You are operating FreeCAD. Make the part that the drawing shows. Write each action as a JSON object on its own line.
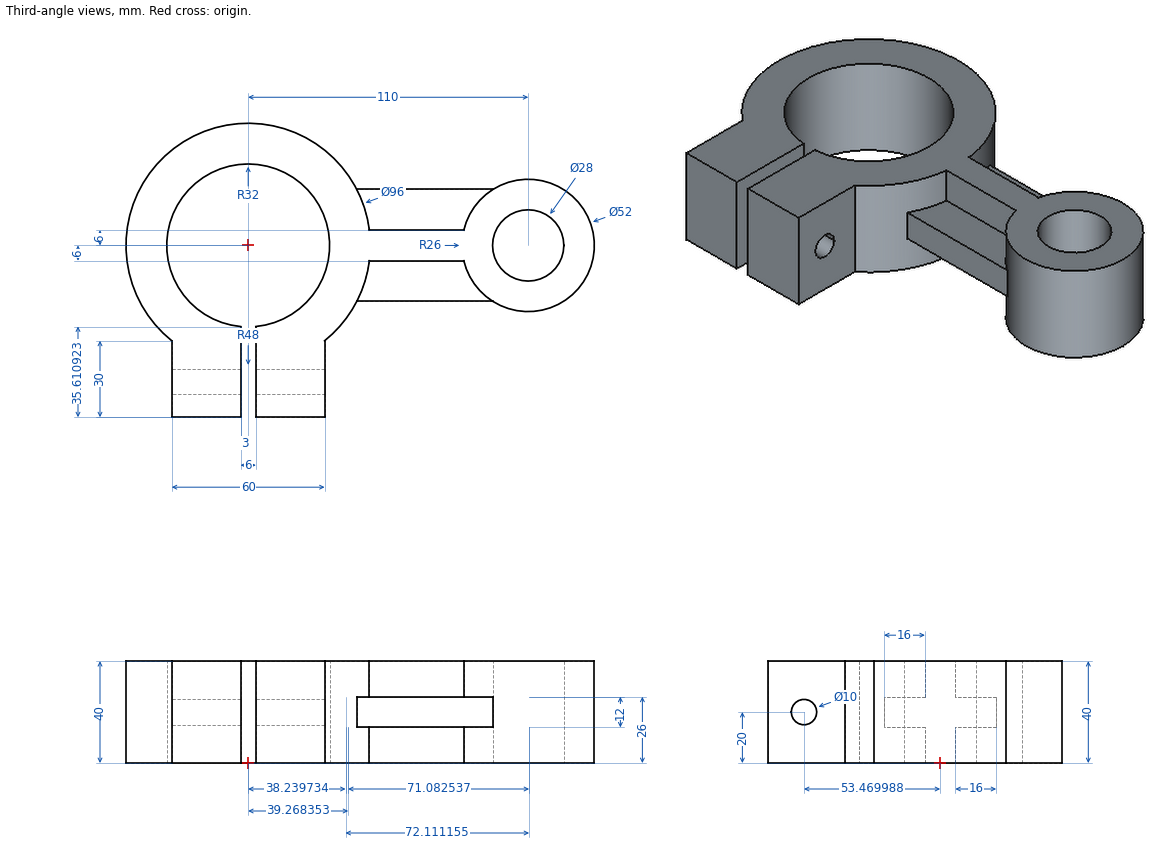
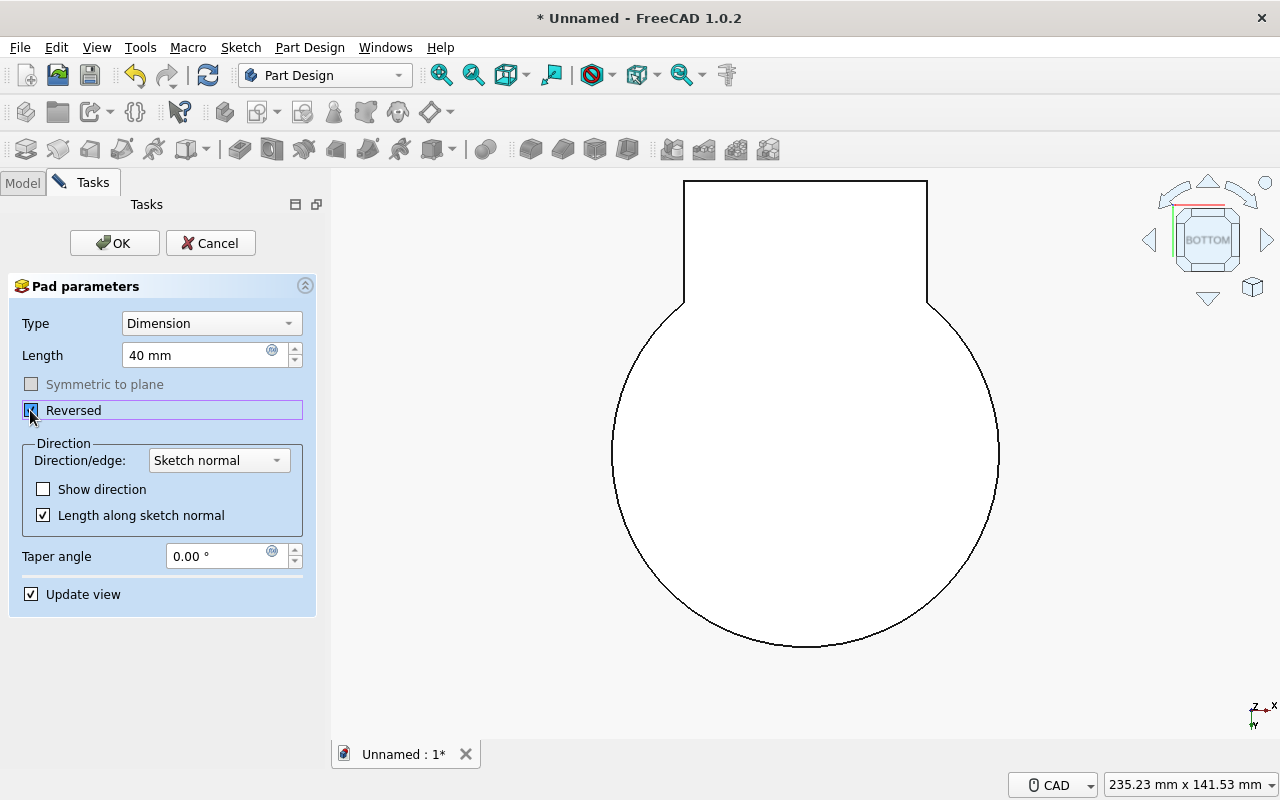
{"action": "left_click", "coordinate": [115, 243]}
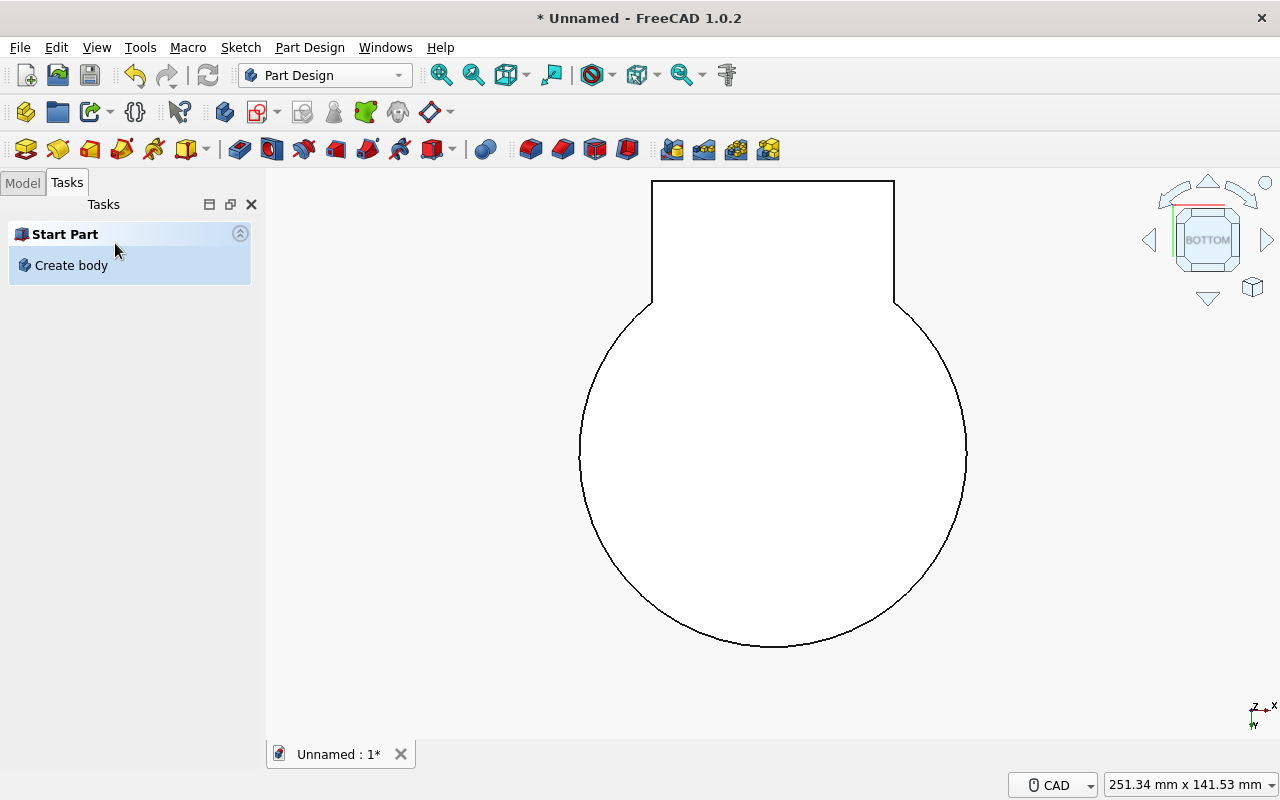
{"action": "key", "text": "0"}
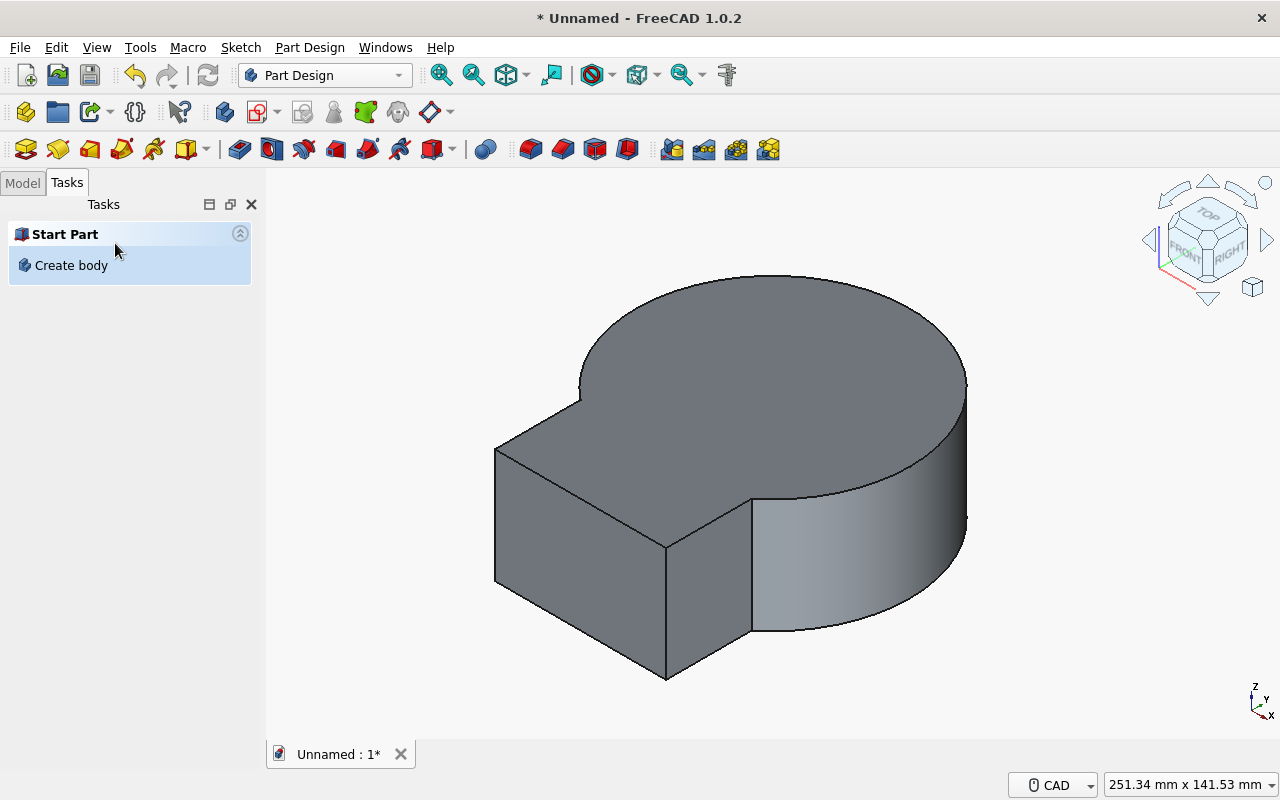
{"action": "left_click", "coordinate": [792, 375]}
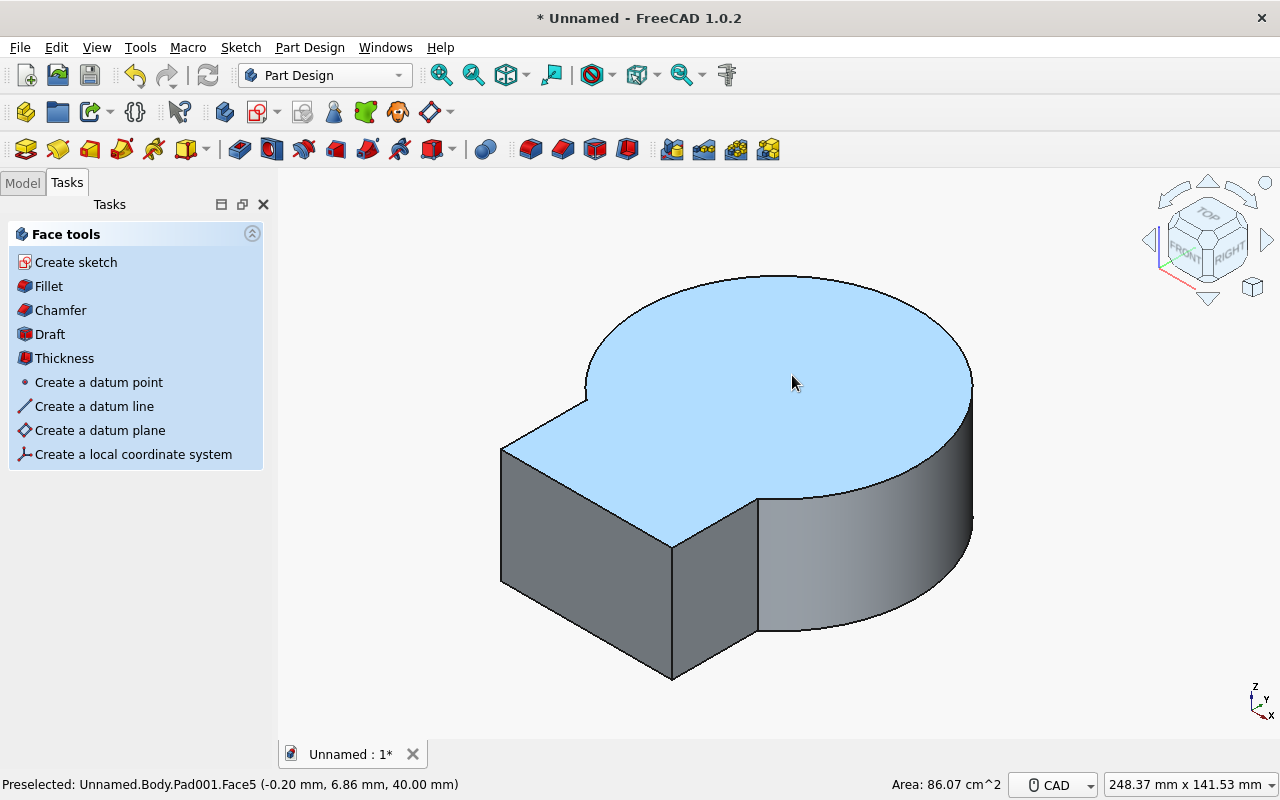
{"action": "left_click", "coordinate": [258, 112]}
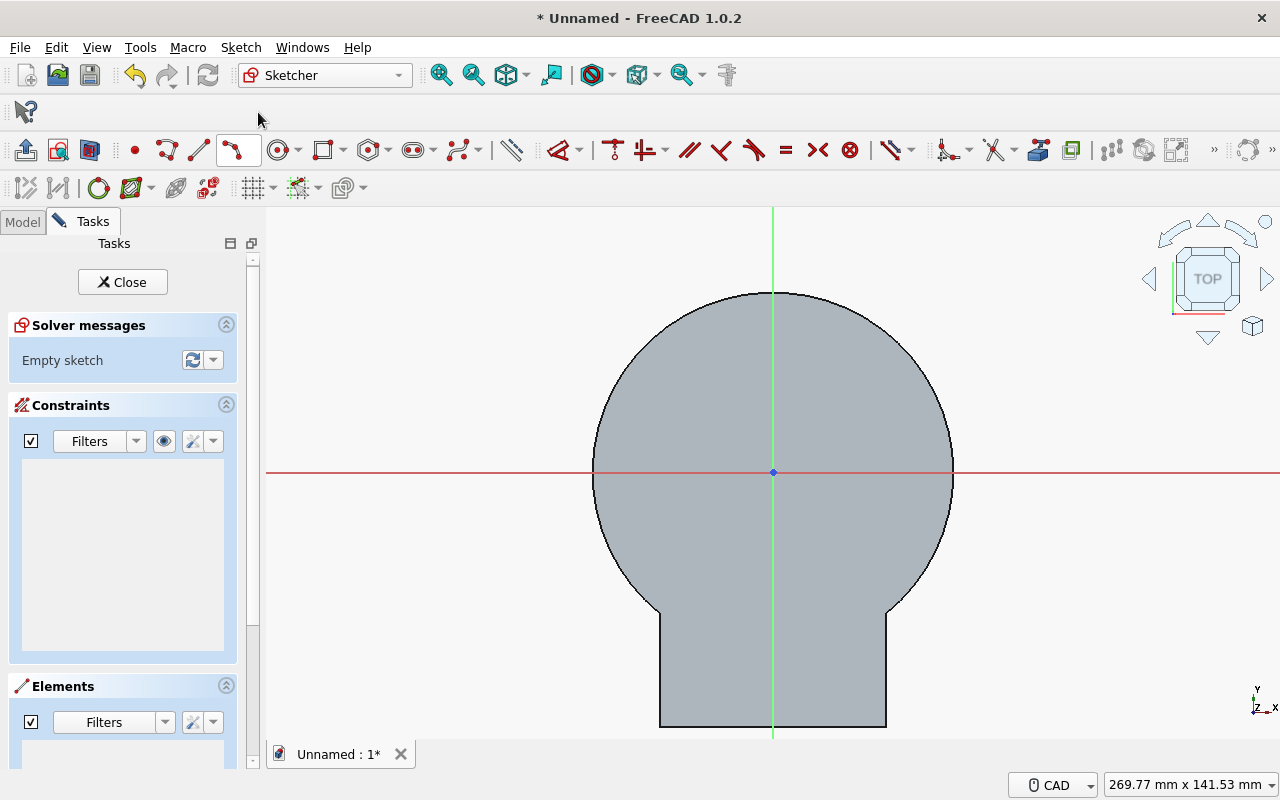
{"action": "scroll", "coordinate": [395, 235], "scroll_direction": "down", "scroll_amount": 1}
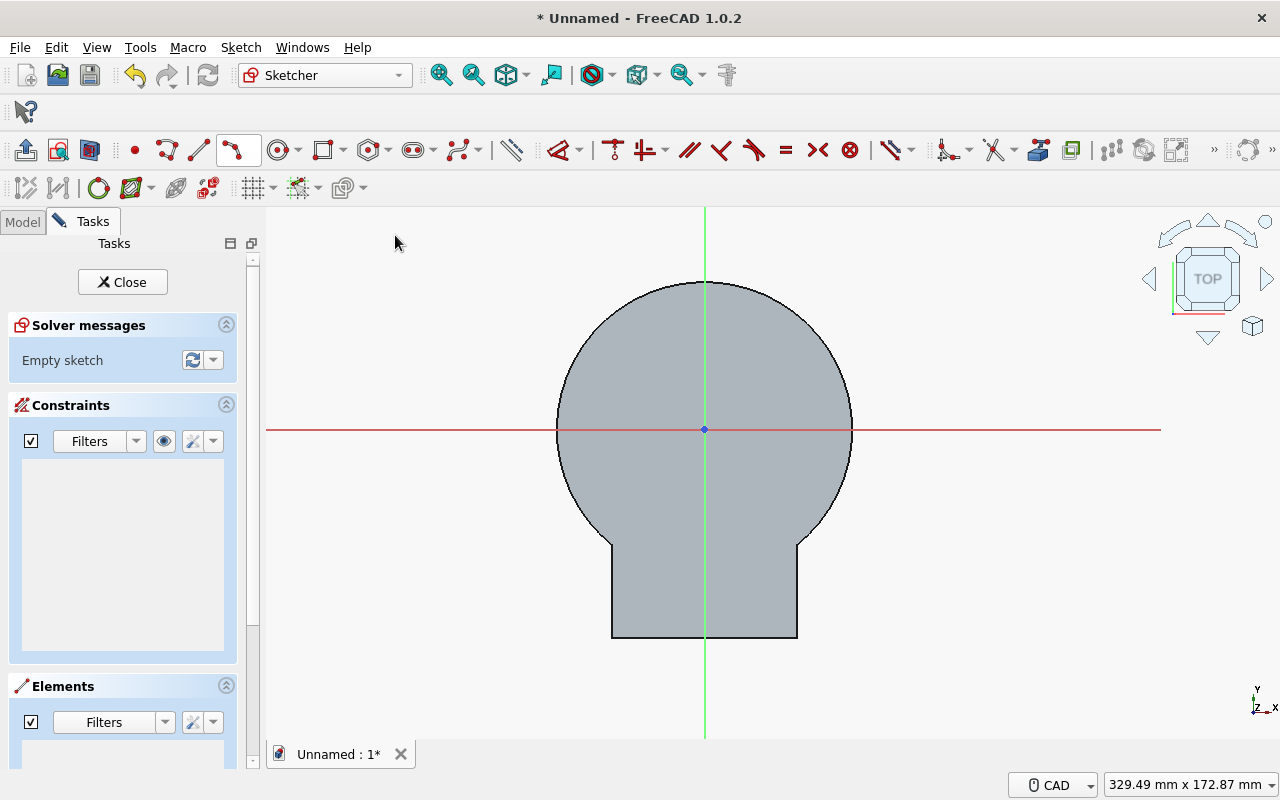
{"action": "left_click", "coordinate": [168, 150]}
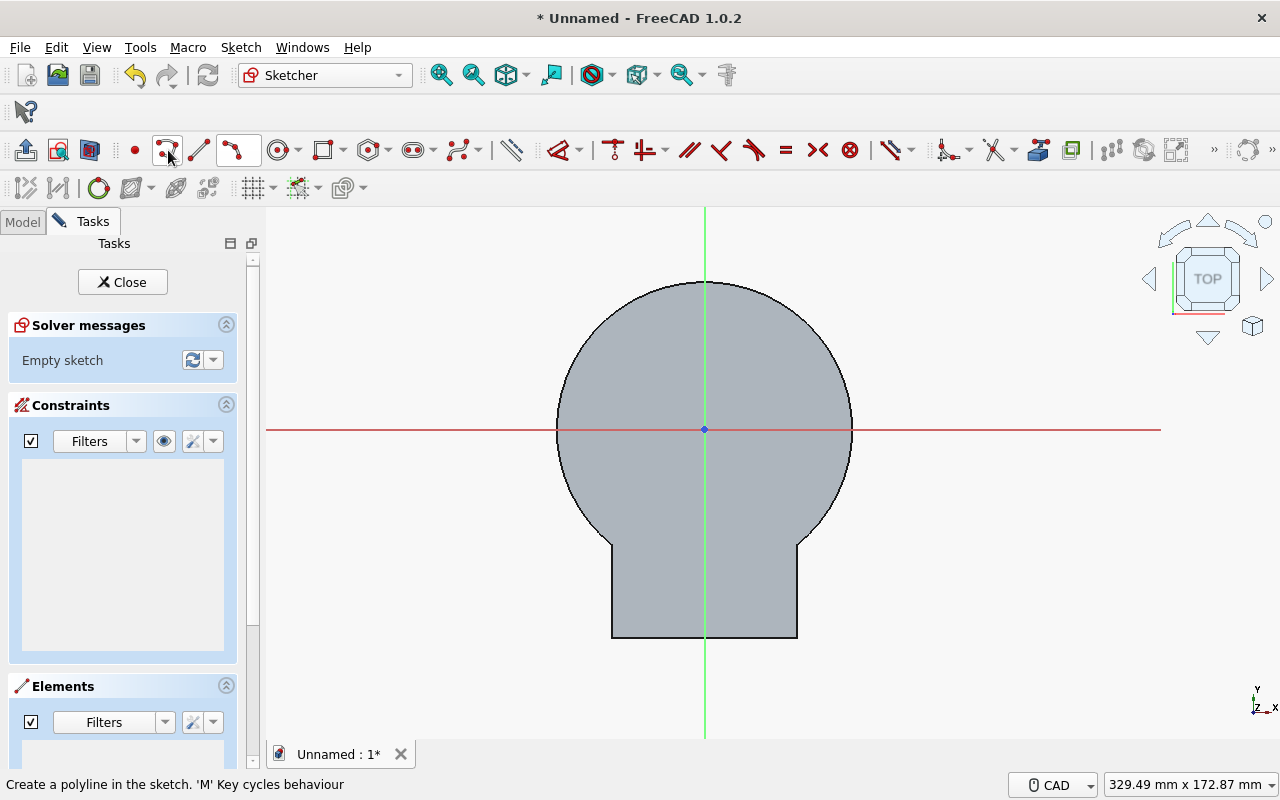
{"action": "scroll", "coordinate": [695, 528], "scroll_direction": "up", "scroll_amount": 3}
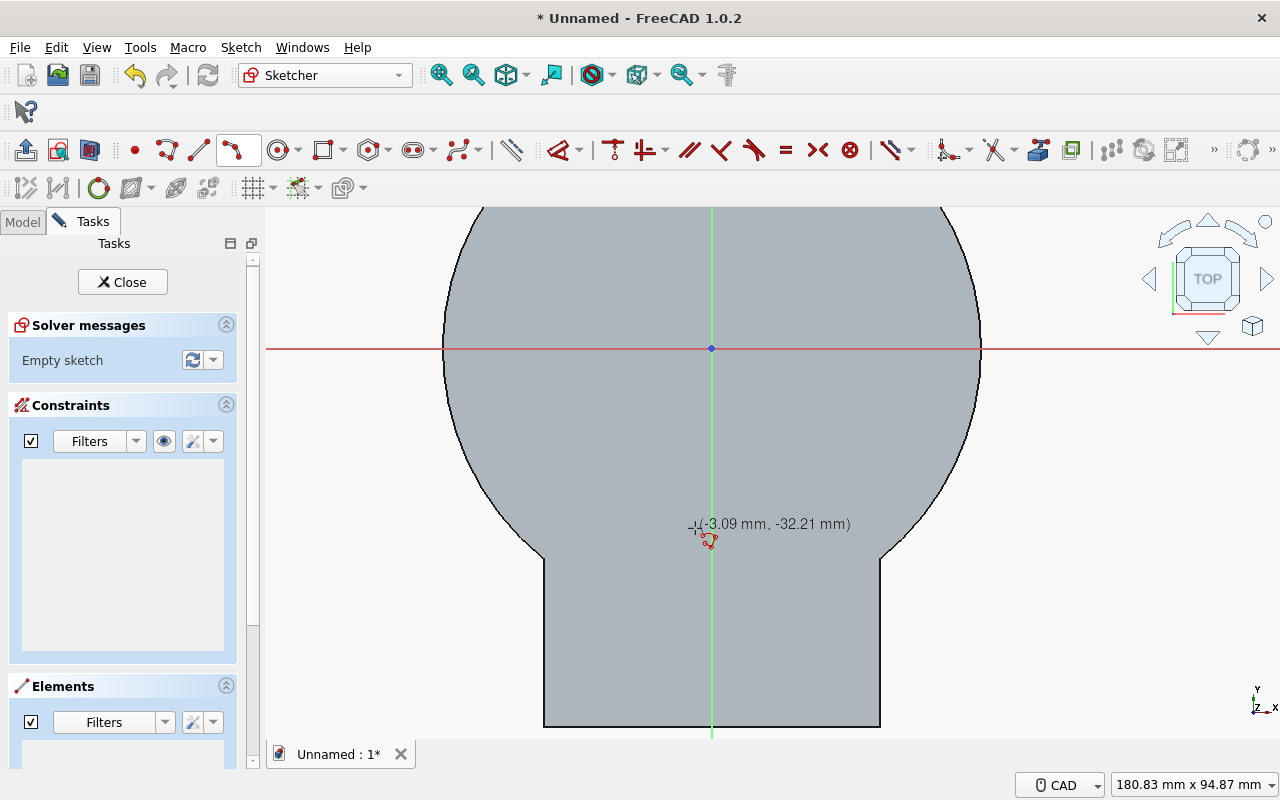
{"action": "left_click", "coordinate": [695, 527]}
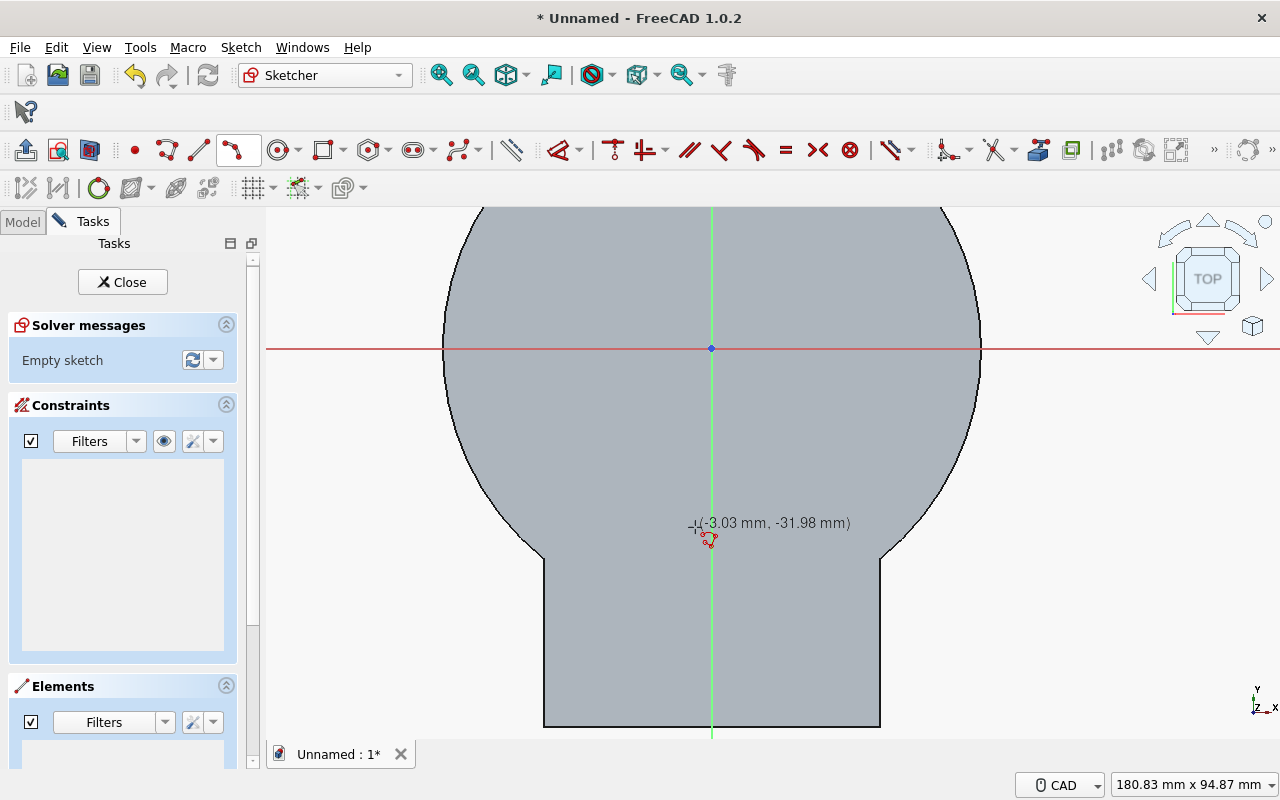
{"action": "scroll", "coordinate": [695, 503], "scroll_direction": "down", "scroll_amount": 3}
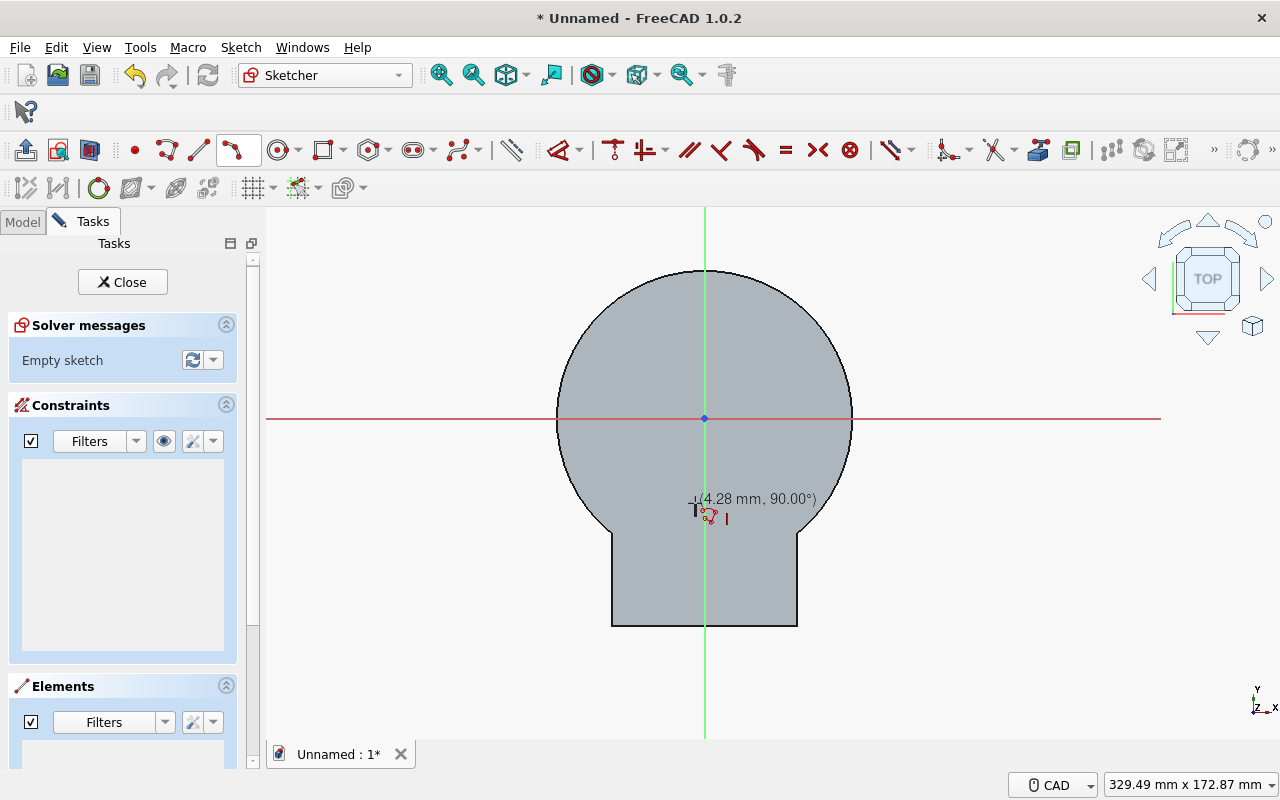
{"action": "scroll", "coordinate": [695, 626], "scroll_direction": "up", "scroll_amount": 3}